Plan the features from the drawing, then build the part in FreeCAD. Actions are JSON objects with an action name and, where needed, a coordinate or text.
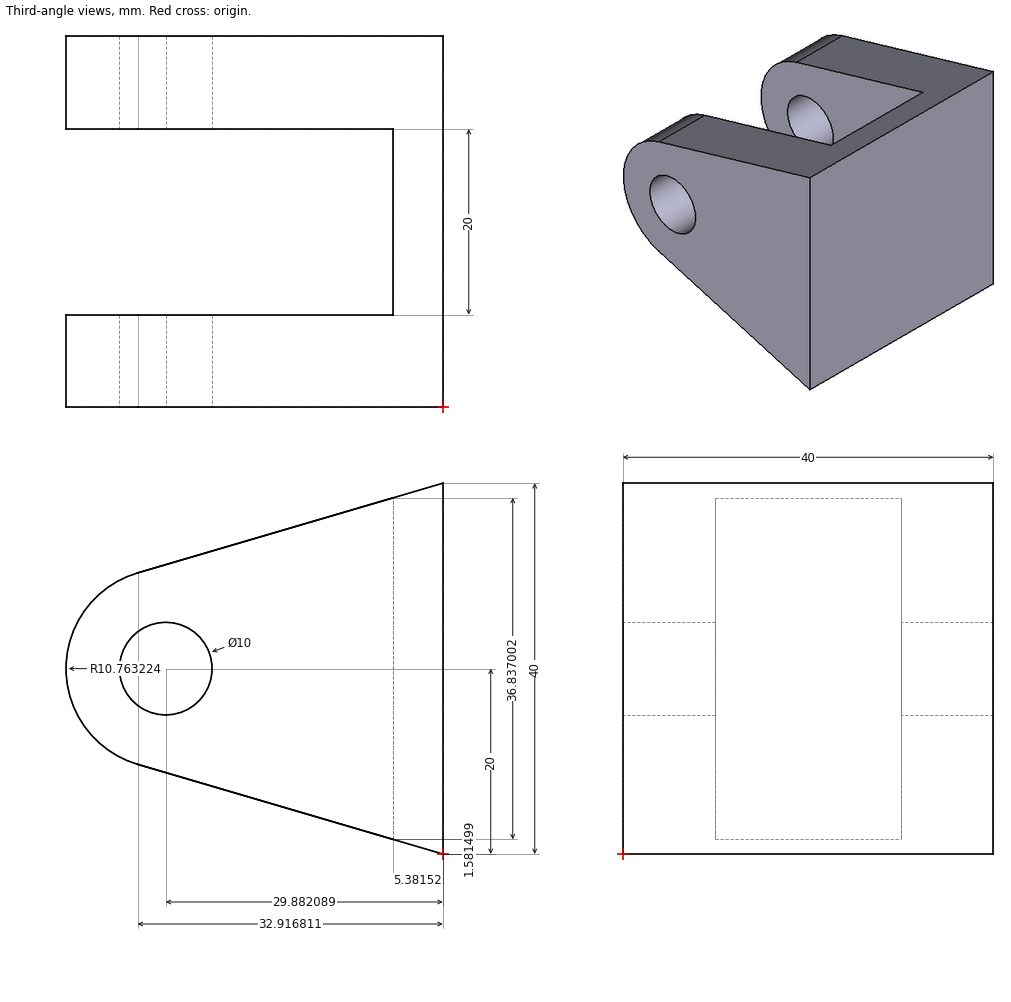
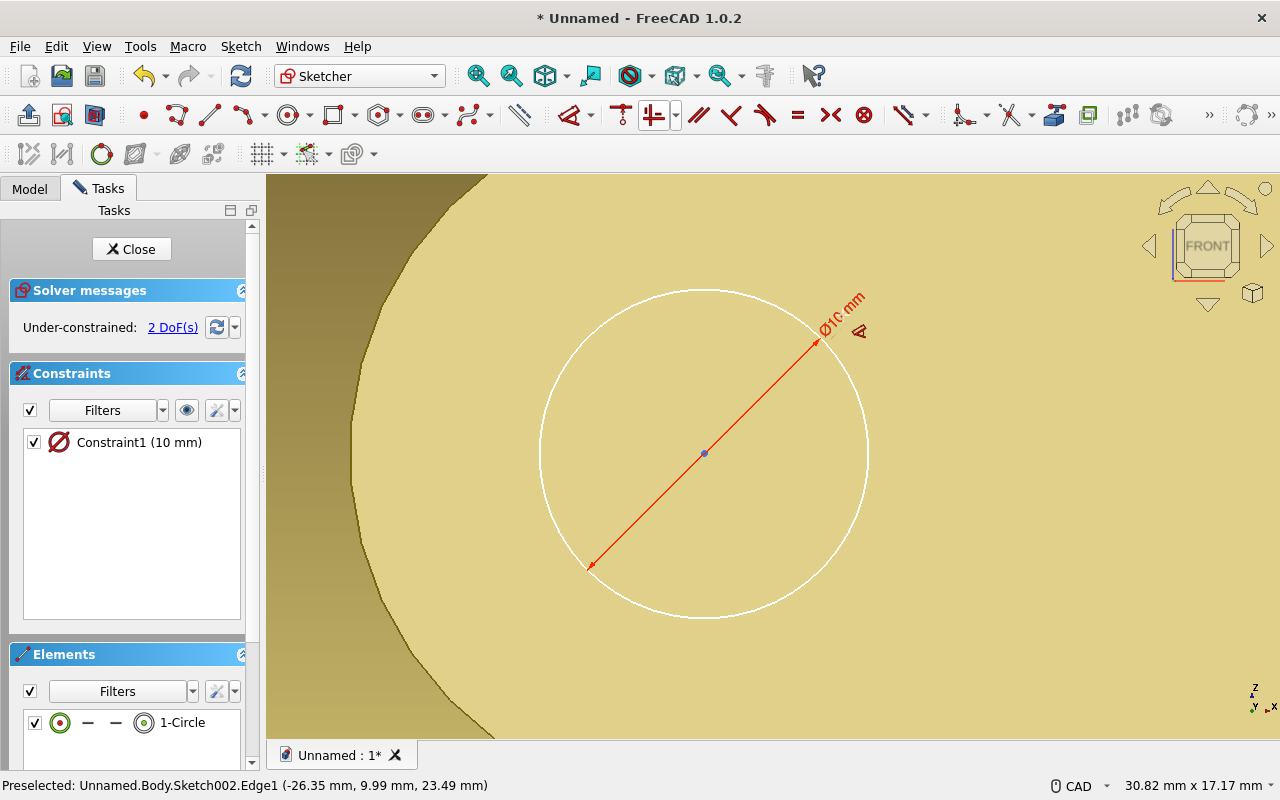
{"action": "left_click", "coordinate": [704, 454]}
{"action": "left_click", "coordinate": [670, 583]}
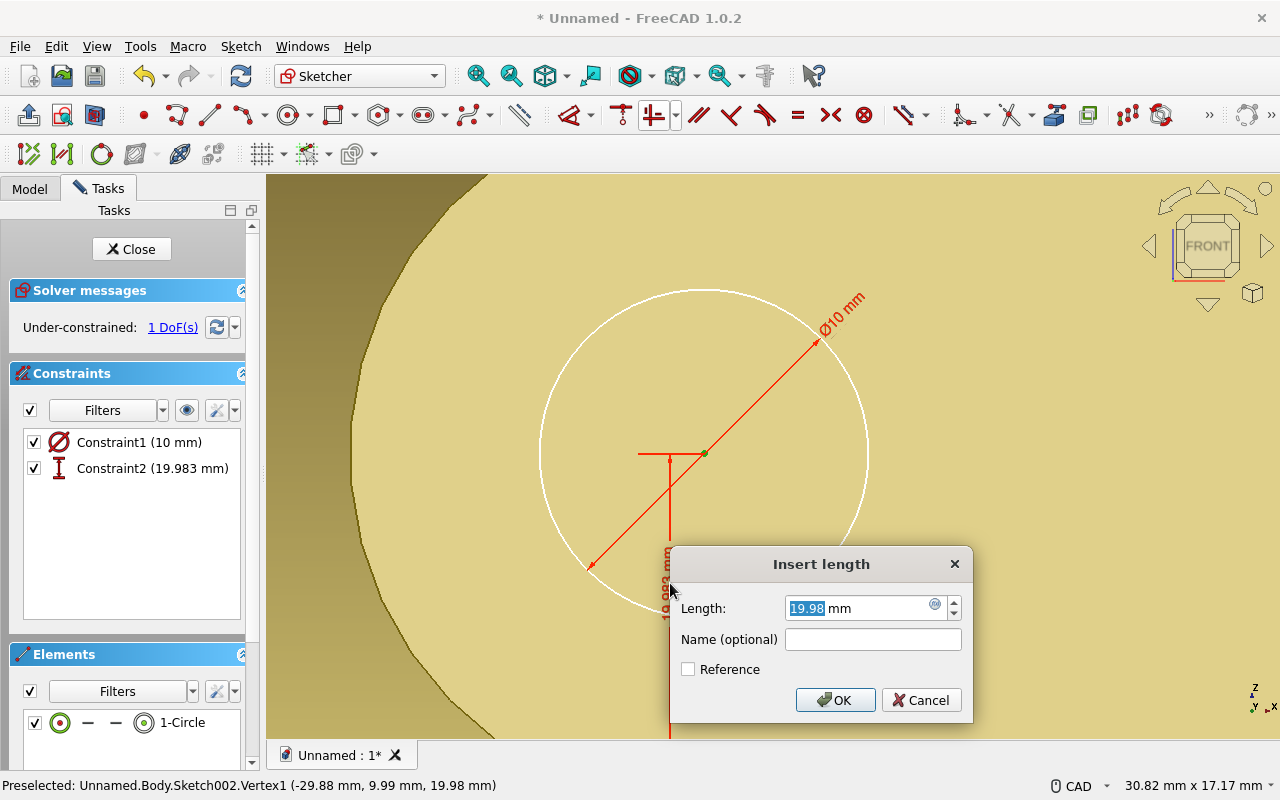
{"action": "type", "text": "20"}
{"action": "key", "text": "Return"}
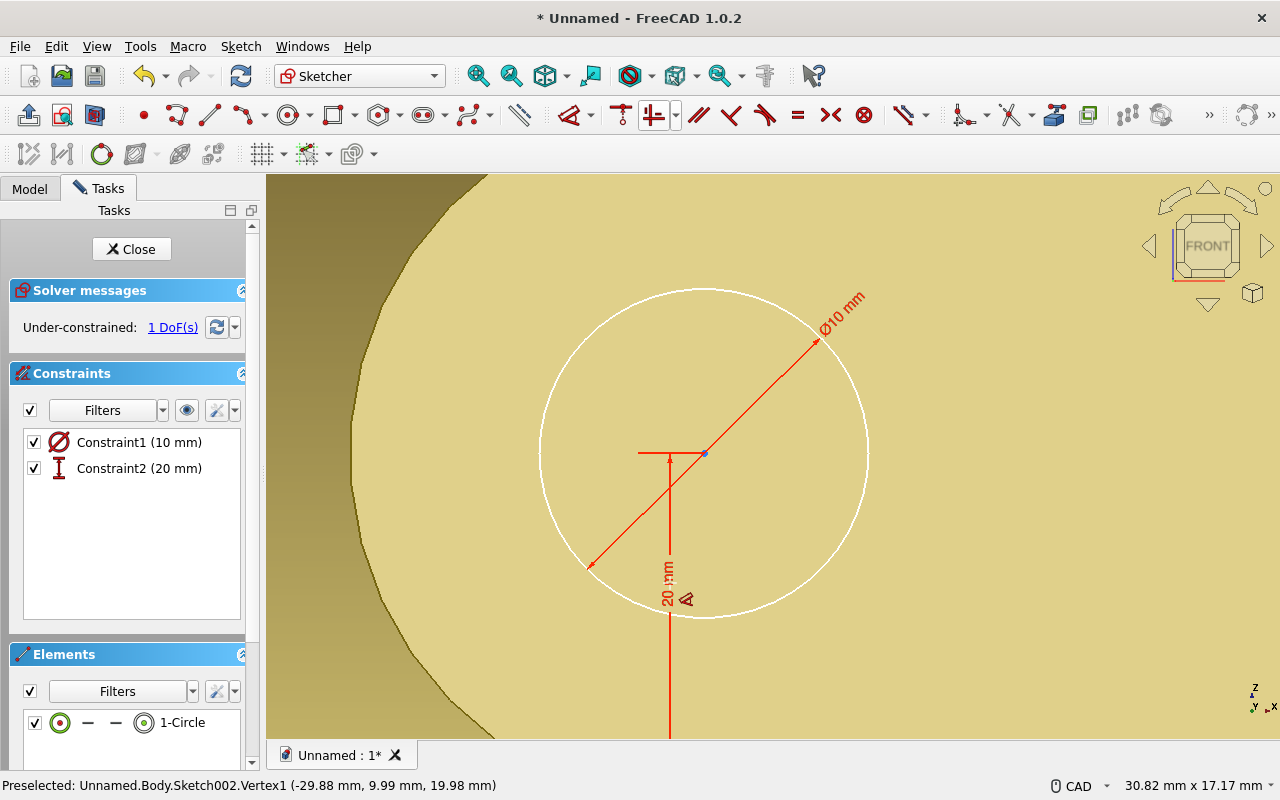
{"action": "left_click", "coordinate": [704, 453]}
{"action": "left_click", "coordinate": [910, 419]}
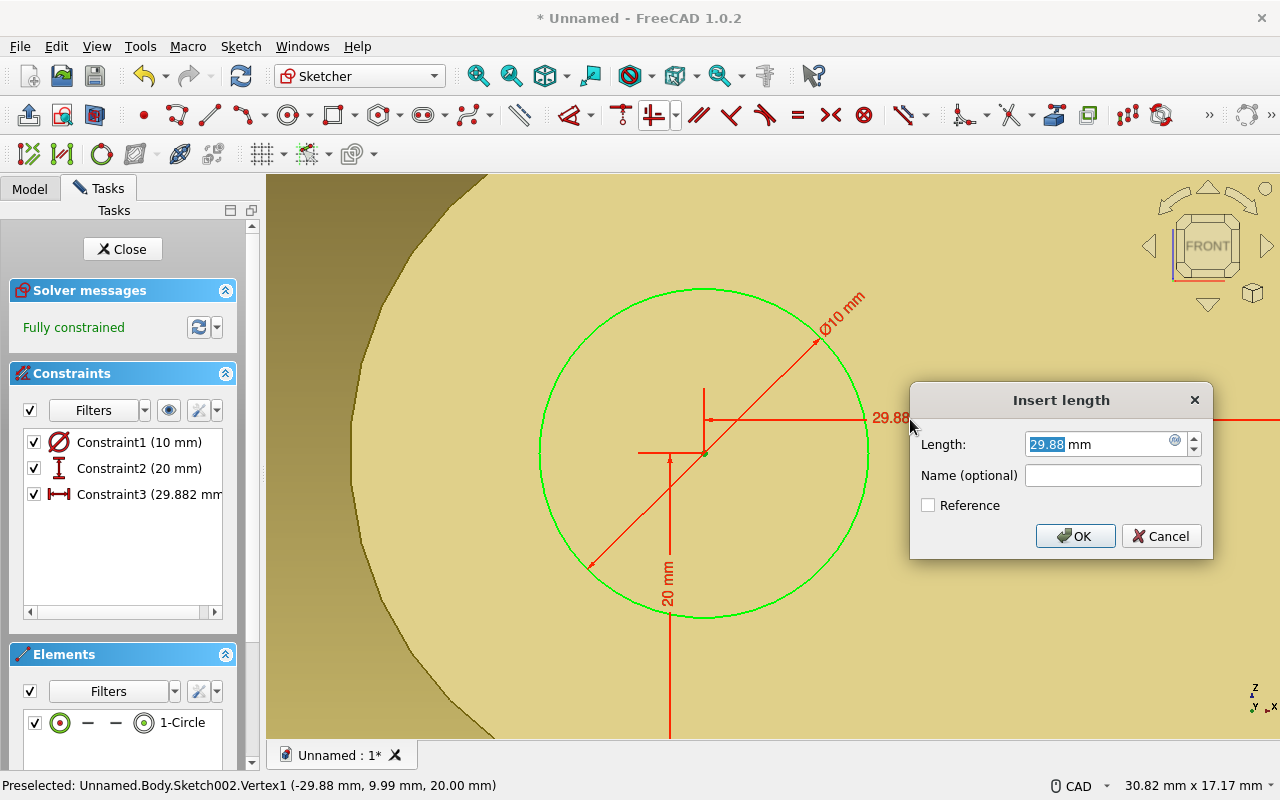
{"action": "type", "text": "29.882089"}
{"action": "key", "text": "Return"}
{"action": "key", "text": "Escape"}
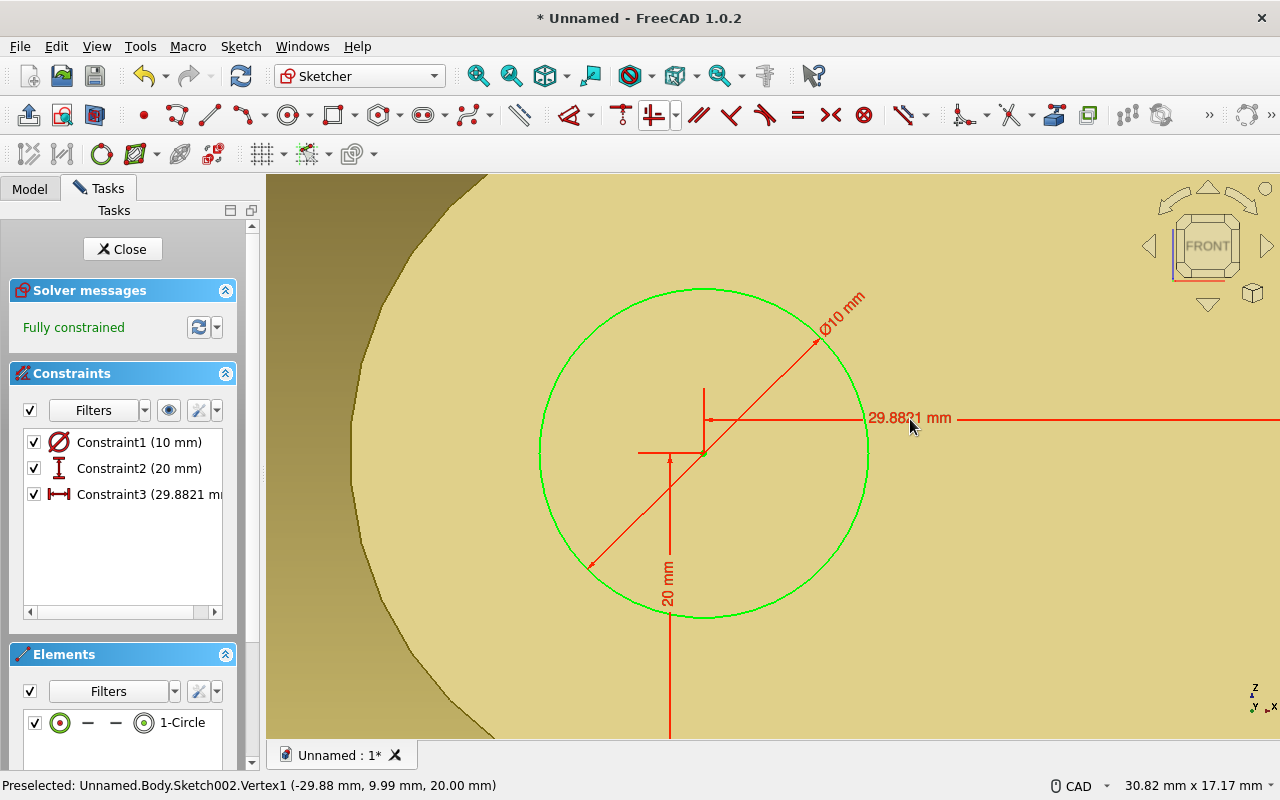
{"action": "left_click", "coordinate": [123, 249]}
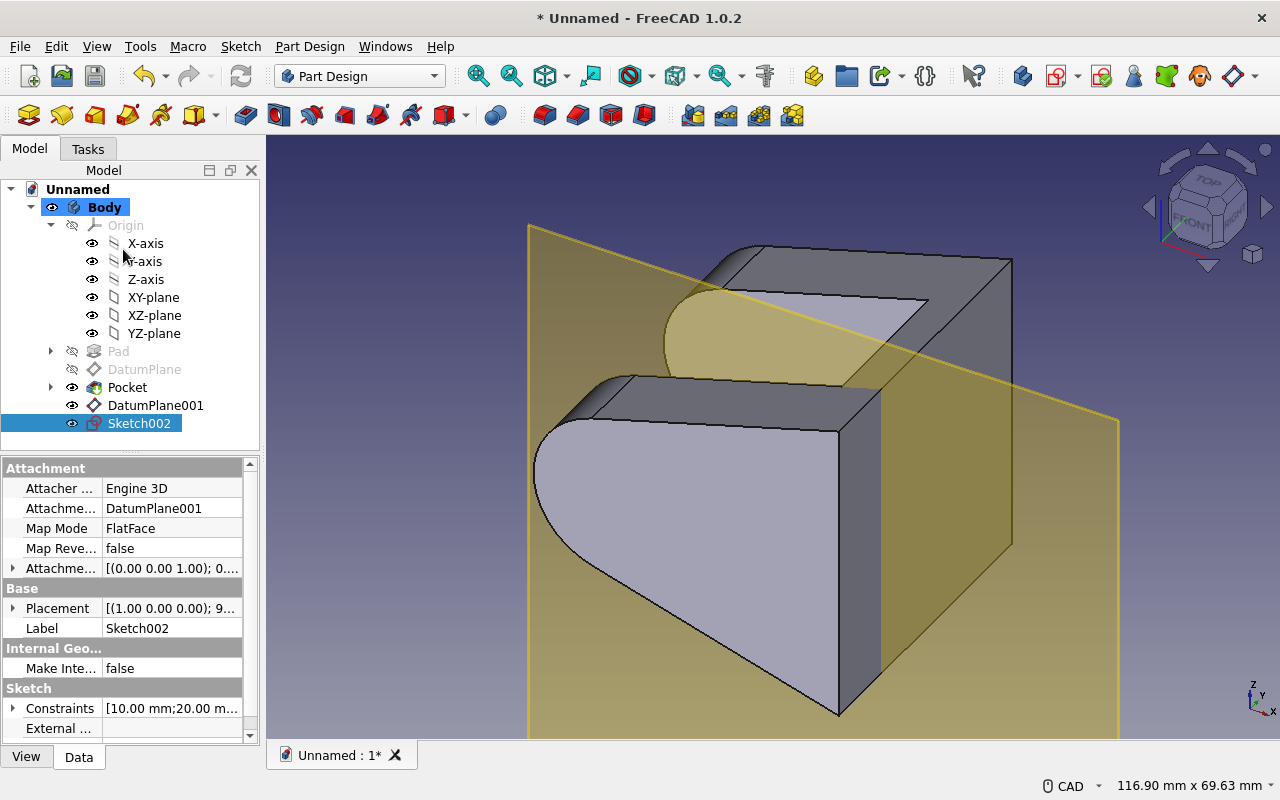
{"action": "left_click", "coordinate": [246, 116]}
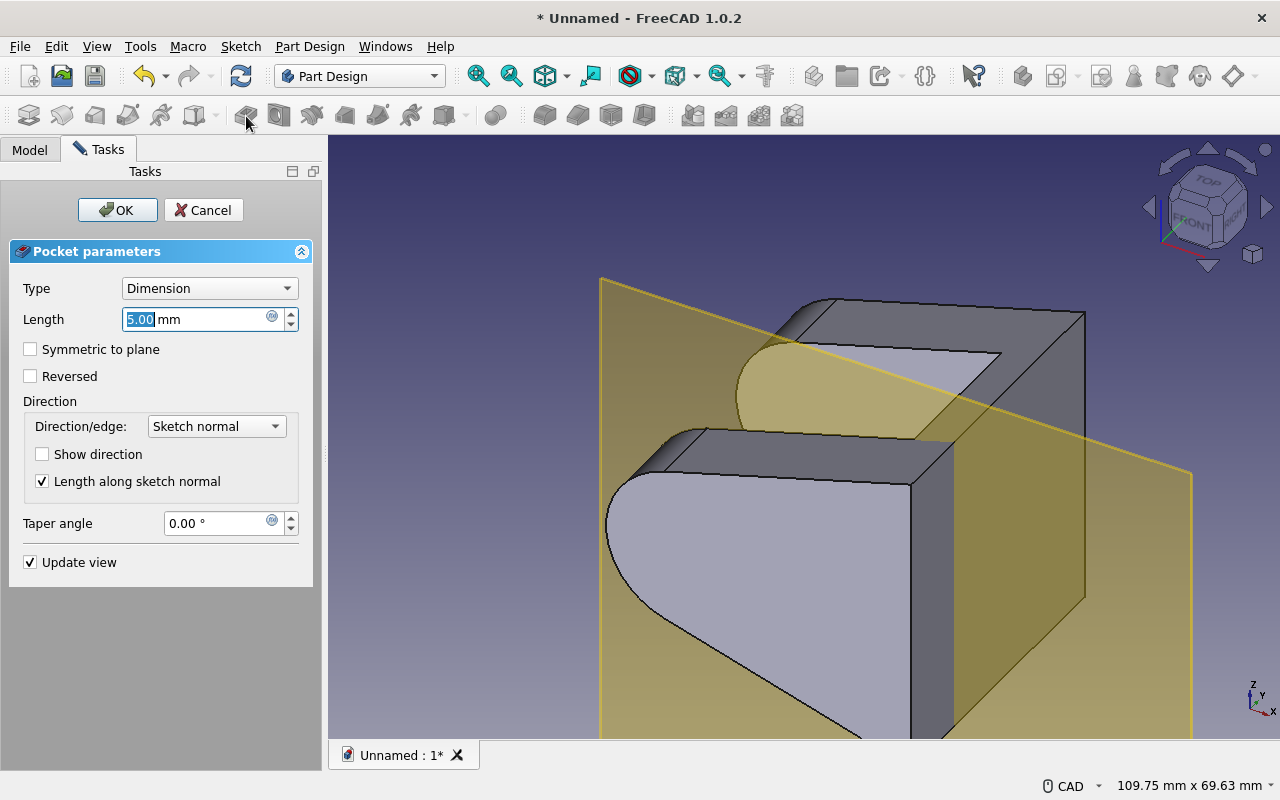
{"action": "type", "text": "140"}
{"action": "key", "text": "Tab"}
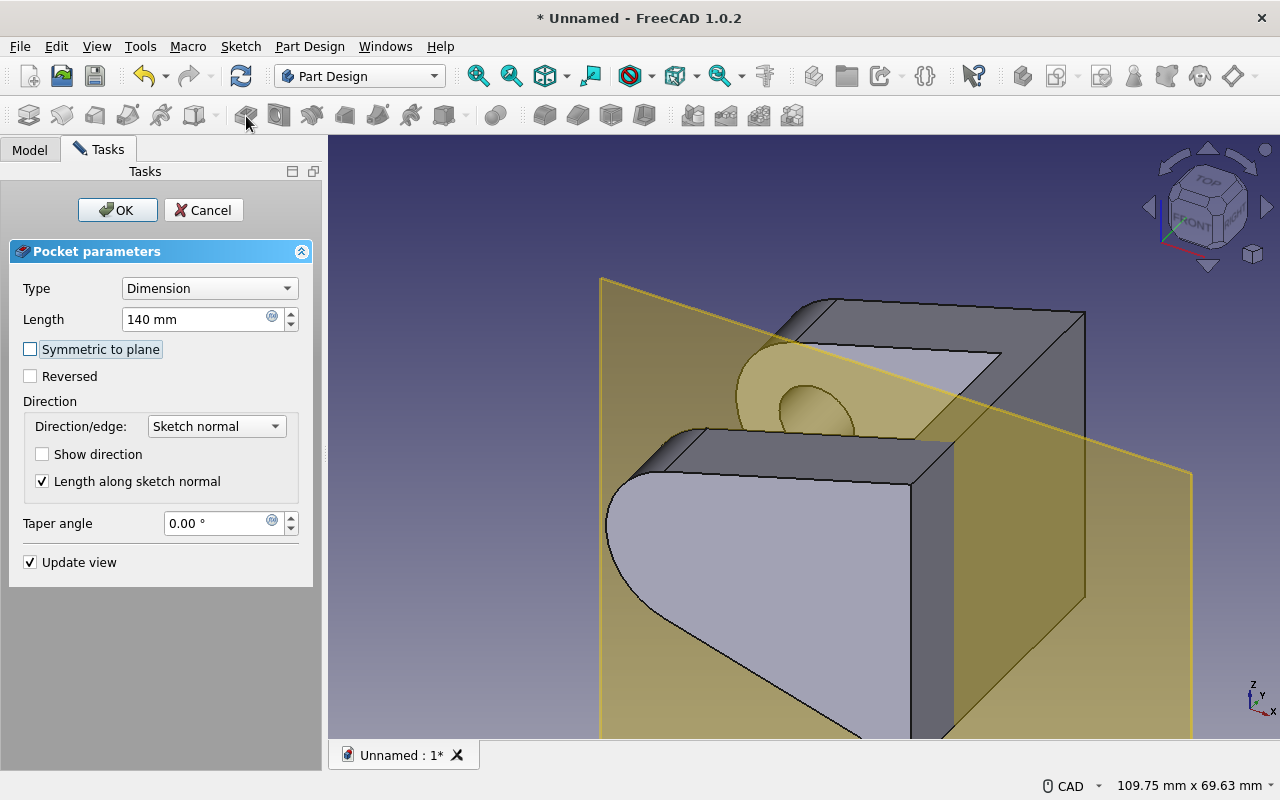
{"action": "left_click", "coordinate": [31, 349]}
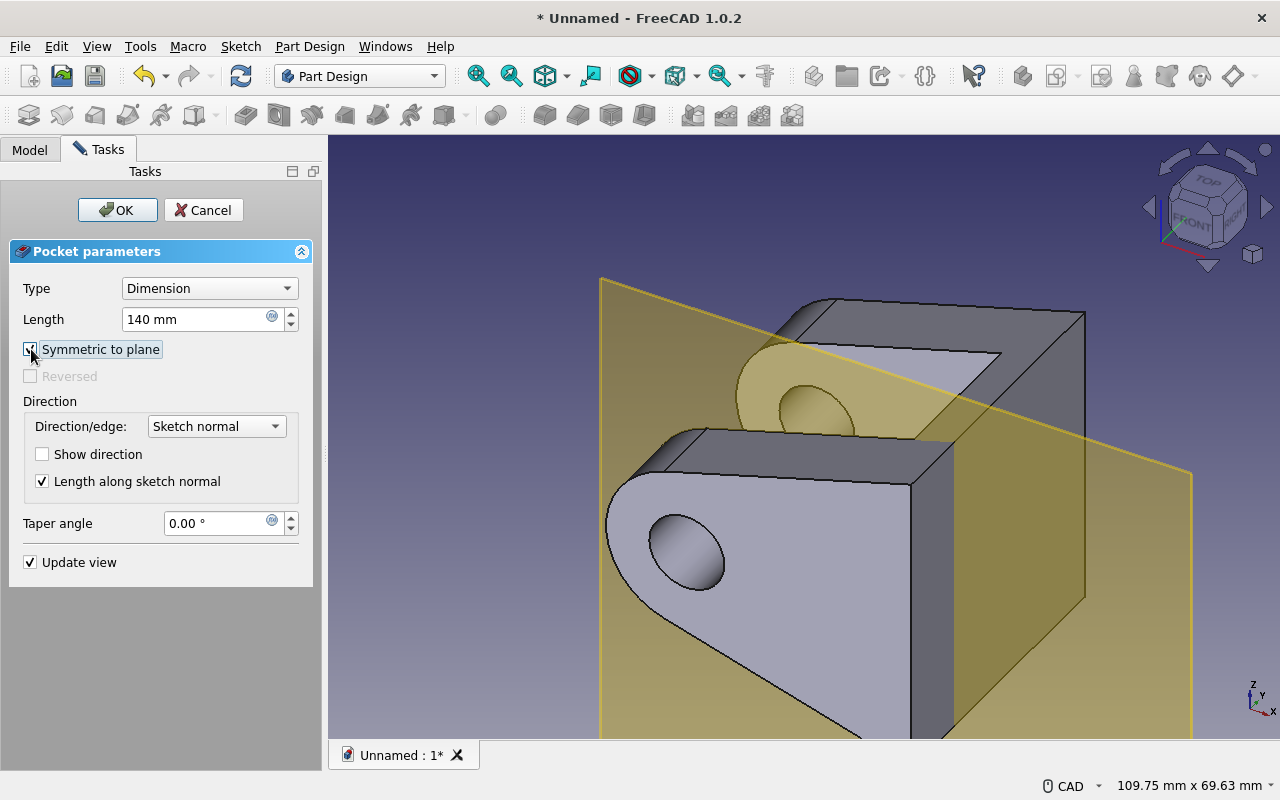
{"action": "left_click", "coordinate": [118, 210]}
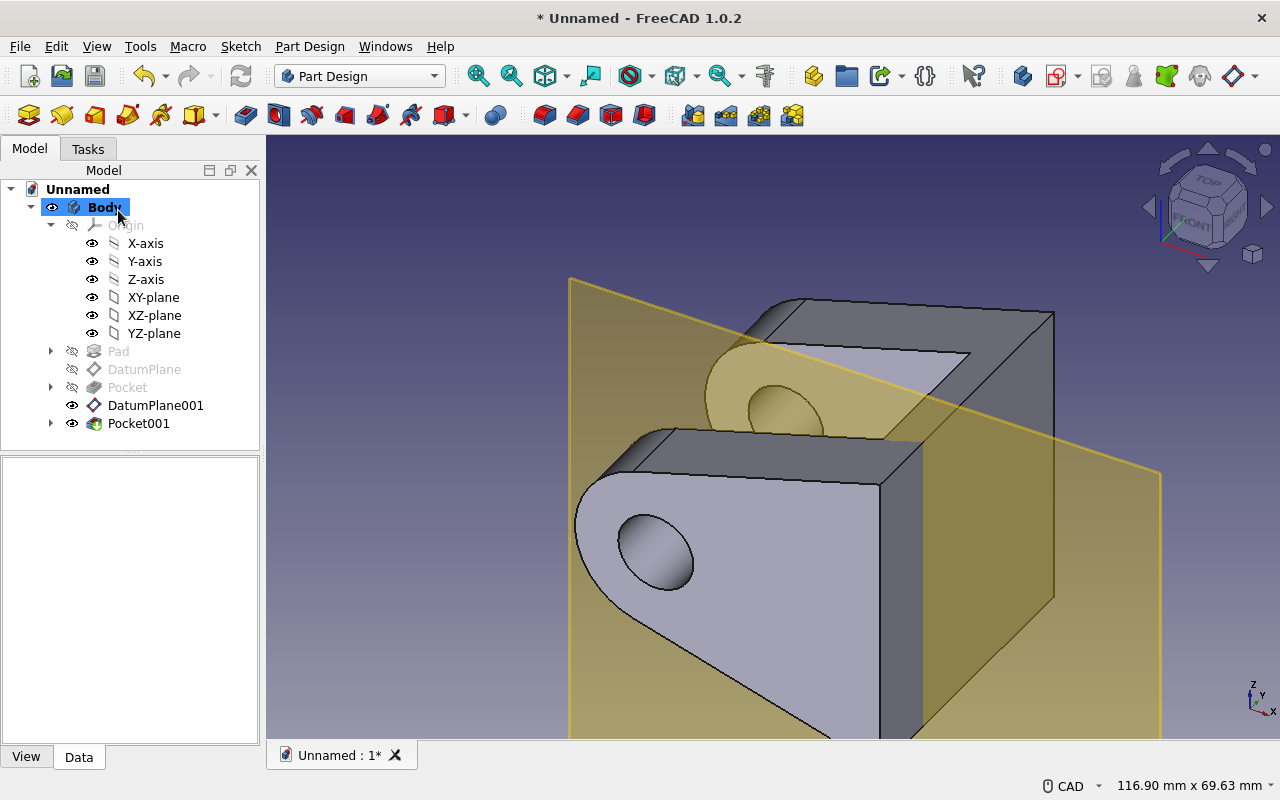
{"action": "left_click", "coordinate": [117, 405]}
{"action": "key", "text": "space"}